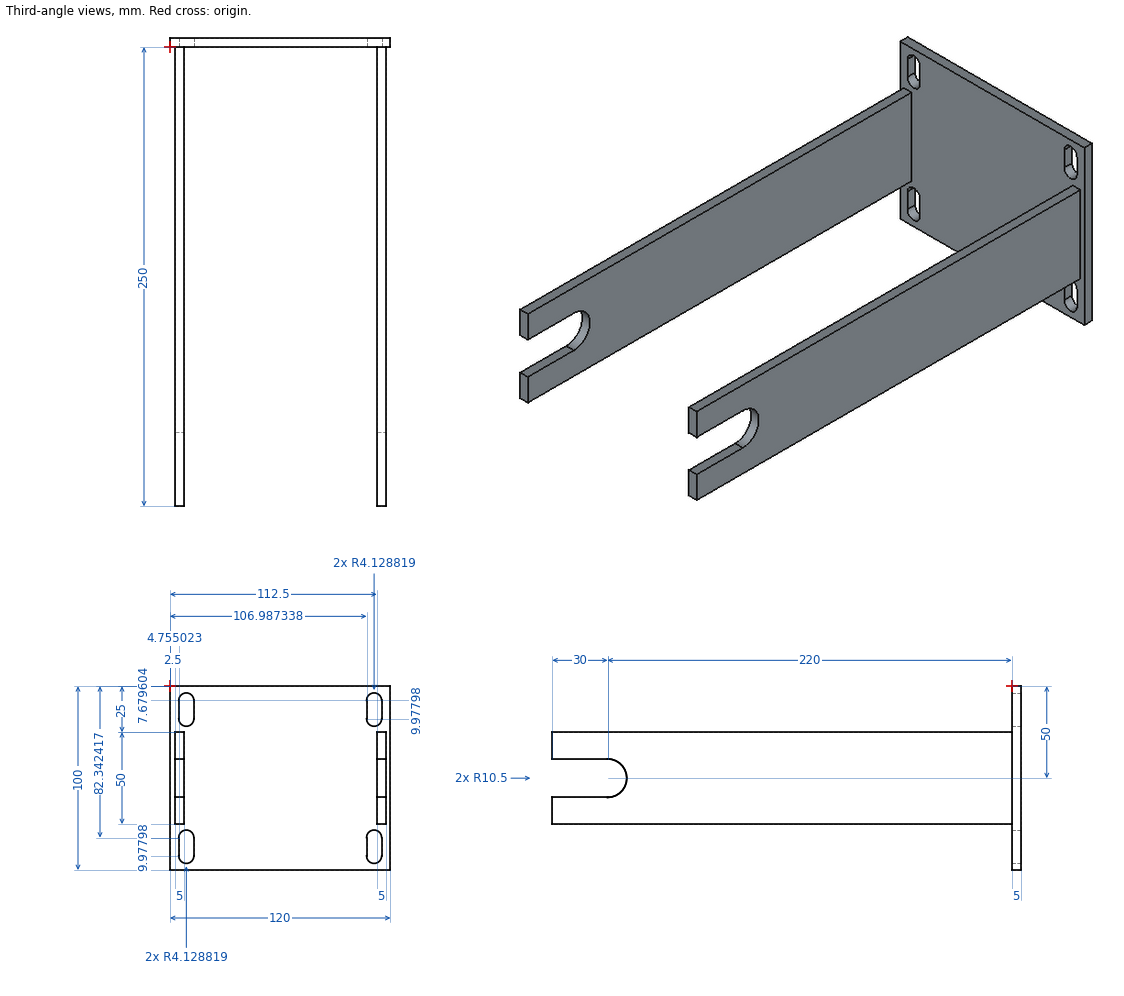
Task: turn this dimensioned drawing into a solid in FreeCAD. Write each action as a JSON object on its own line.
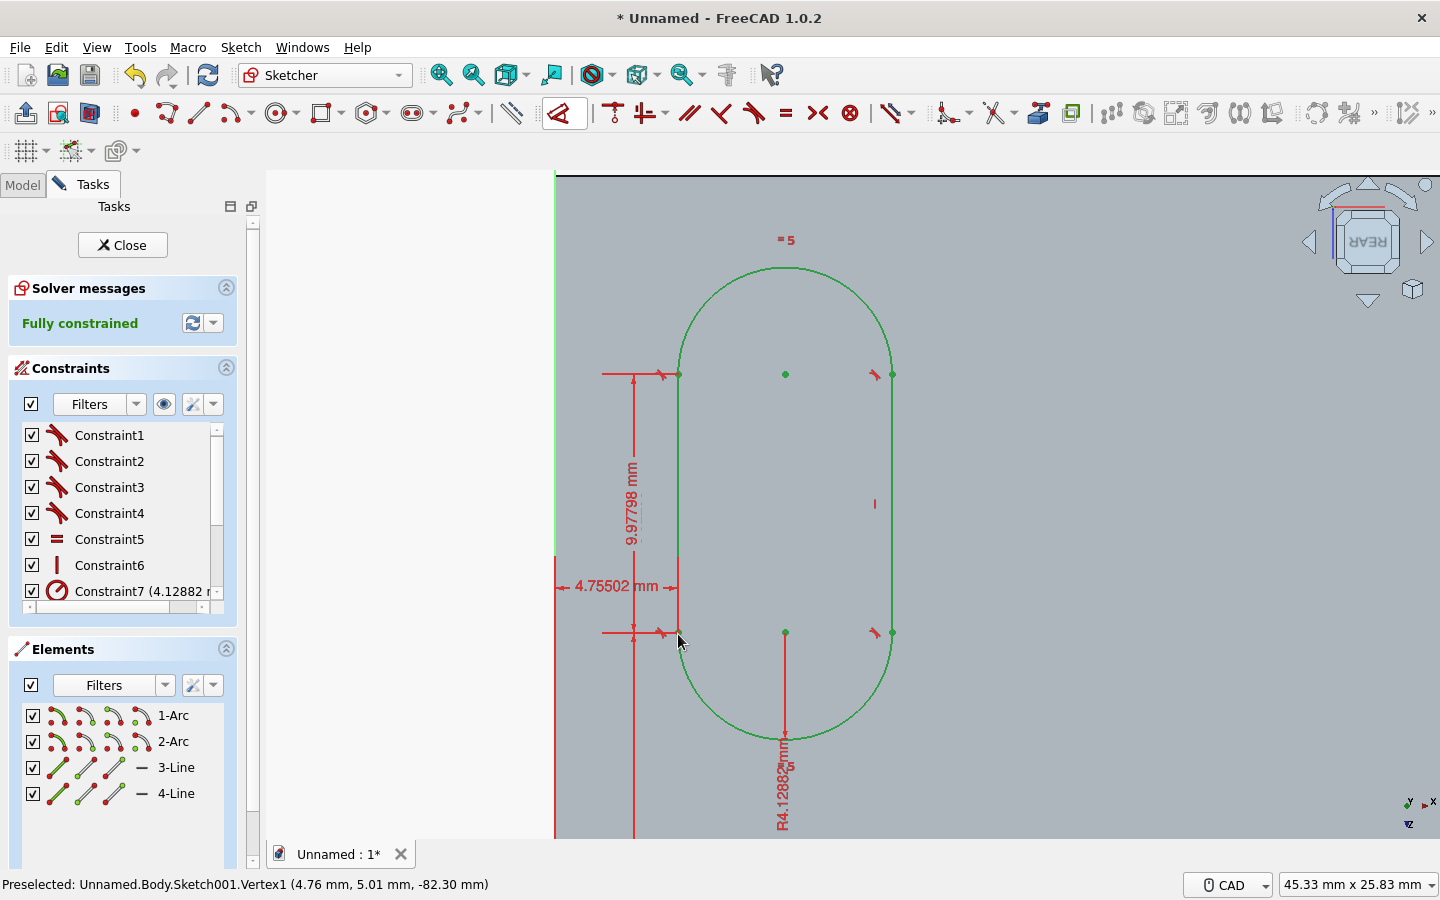
{"action": "left_click", "coordinate": [123, 245]}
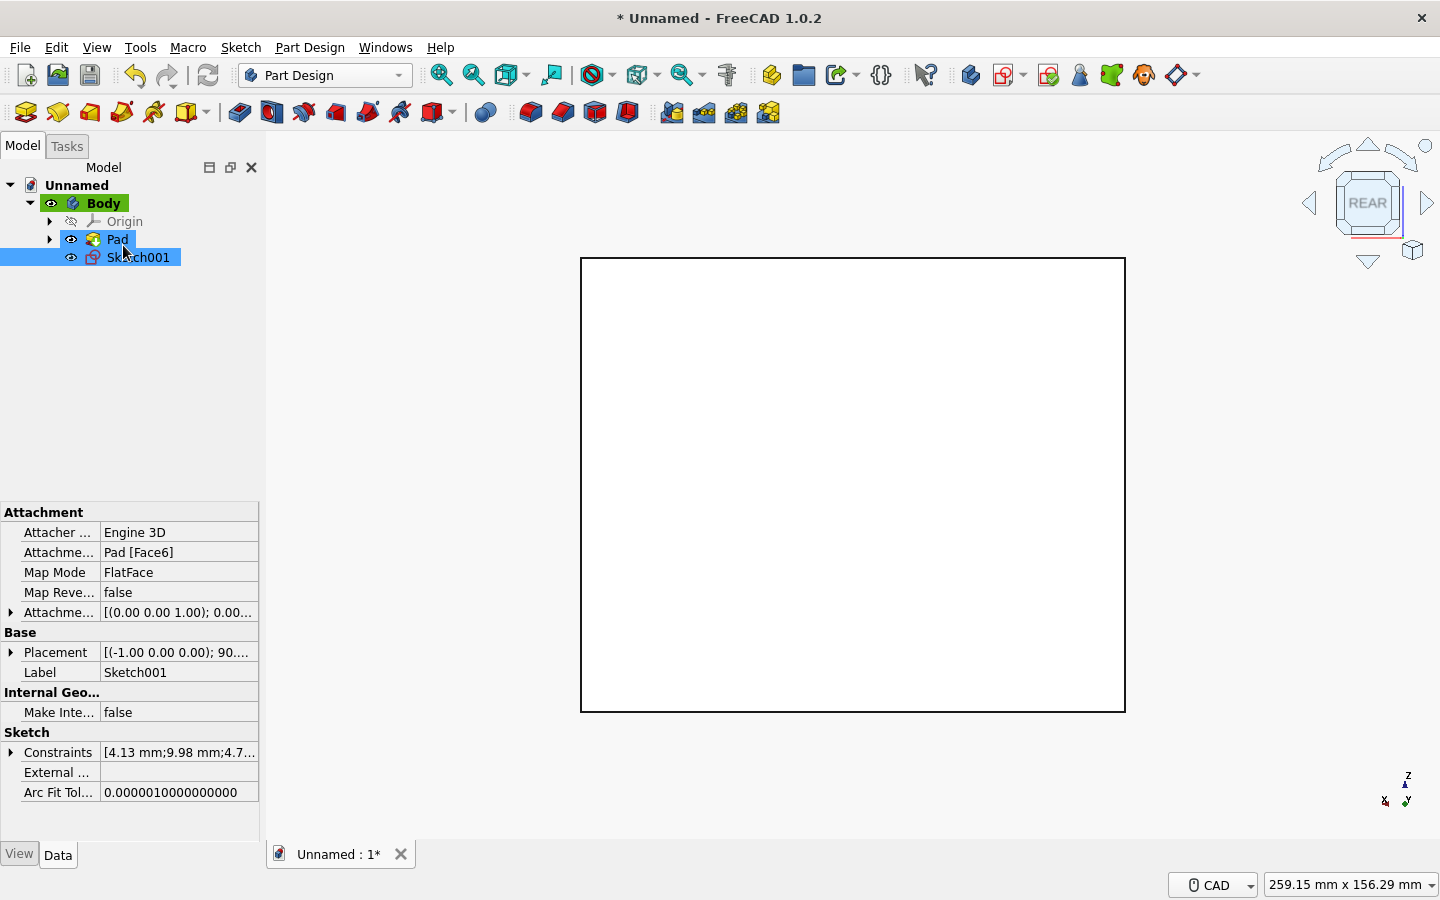
{"action": "left_click", "coordinate": [240, 112]}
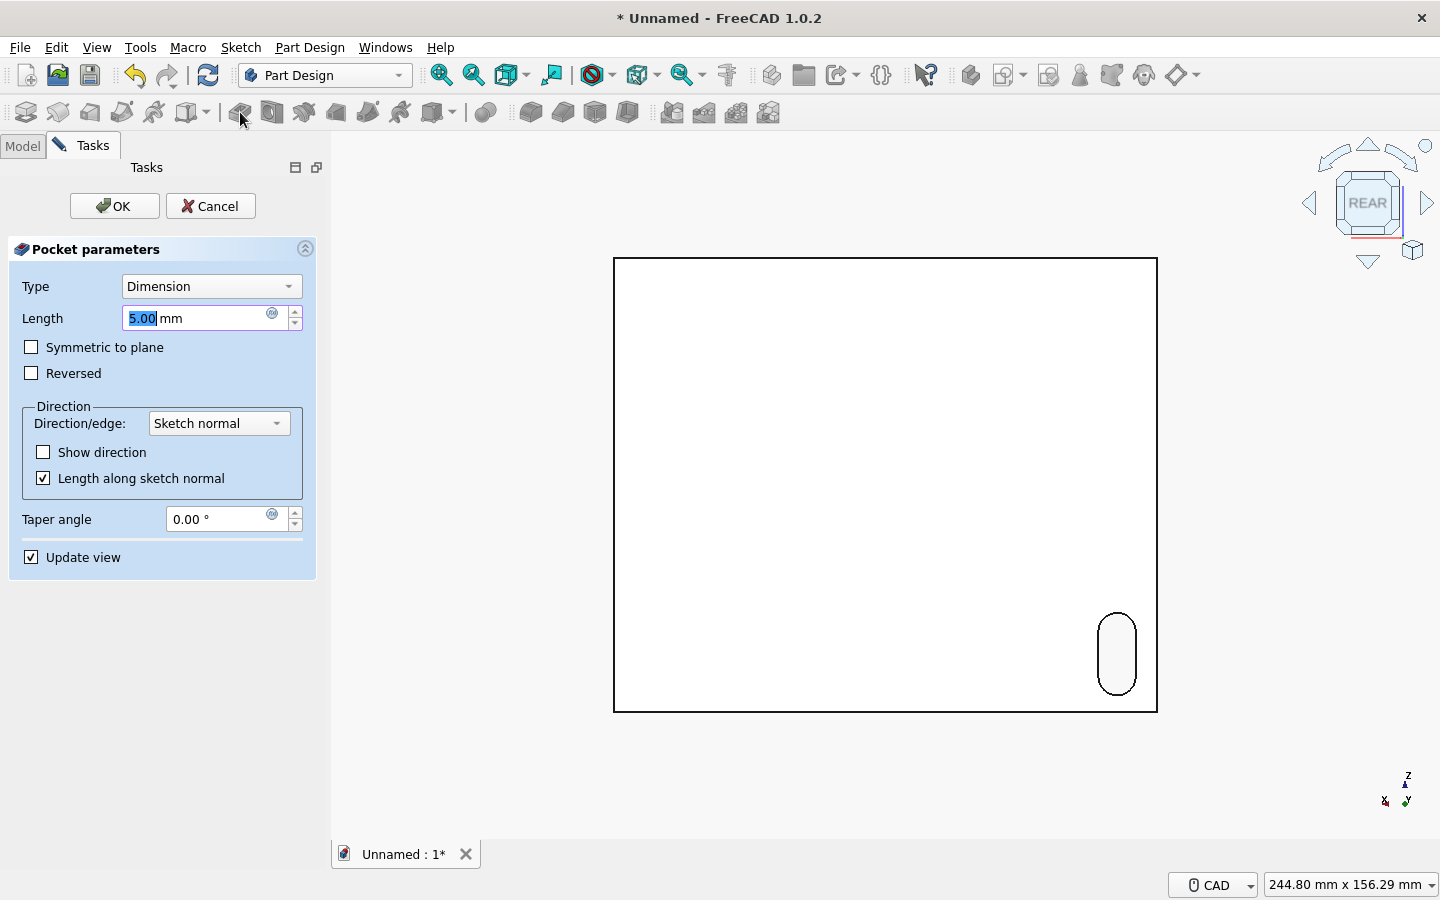
{"action": "left_click", "coordinate": [212, 286]}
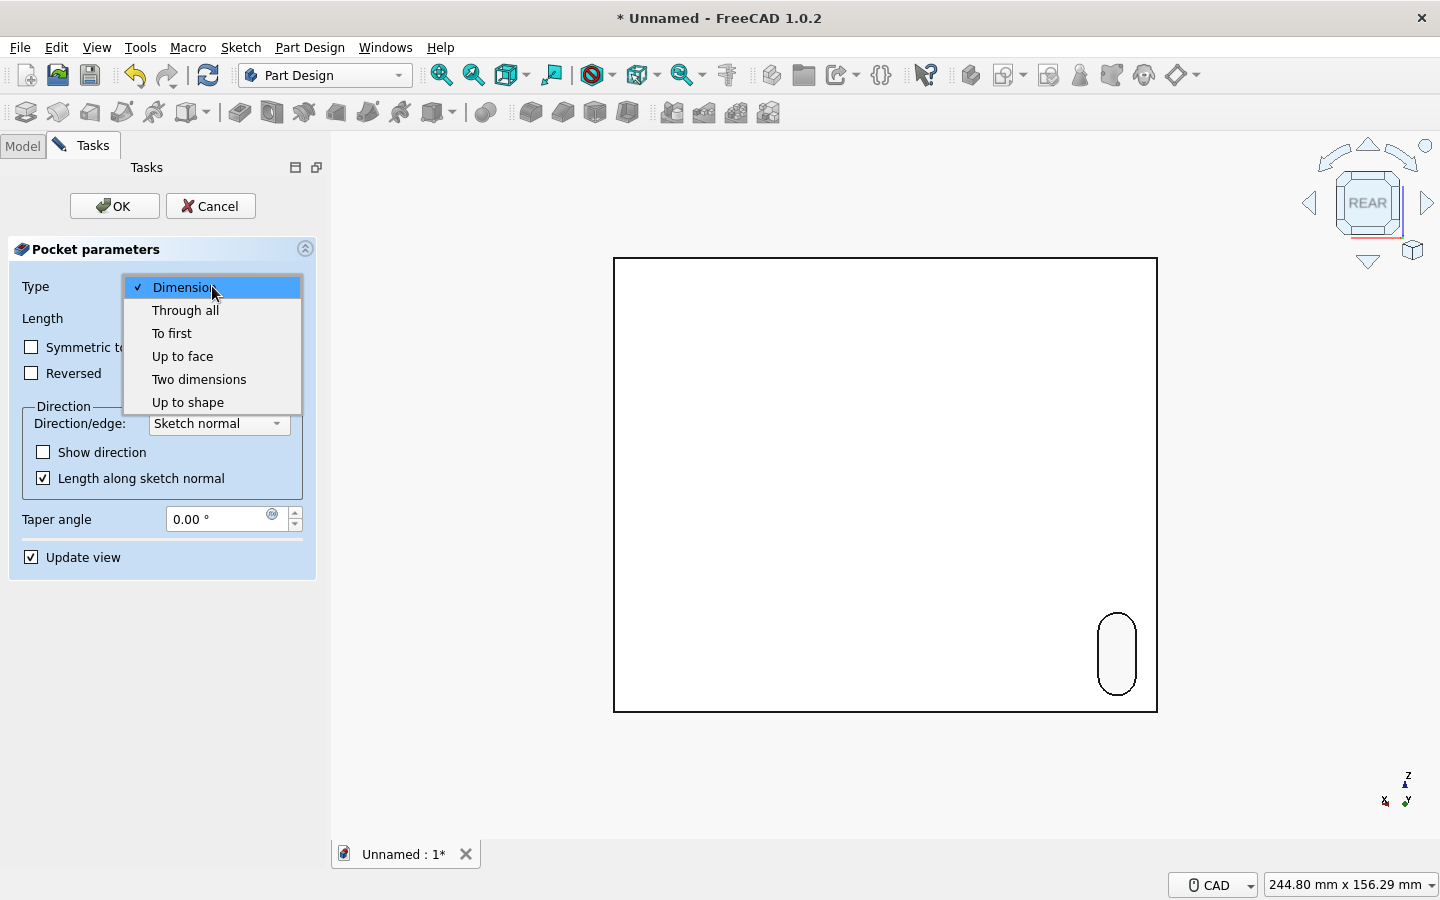
{"action": "left_click", "coordinate": [212, 310]}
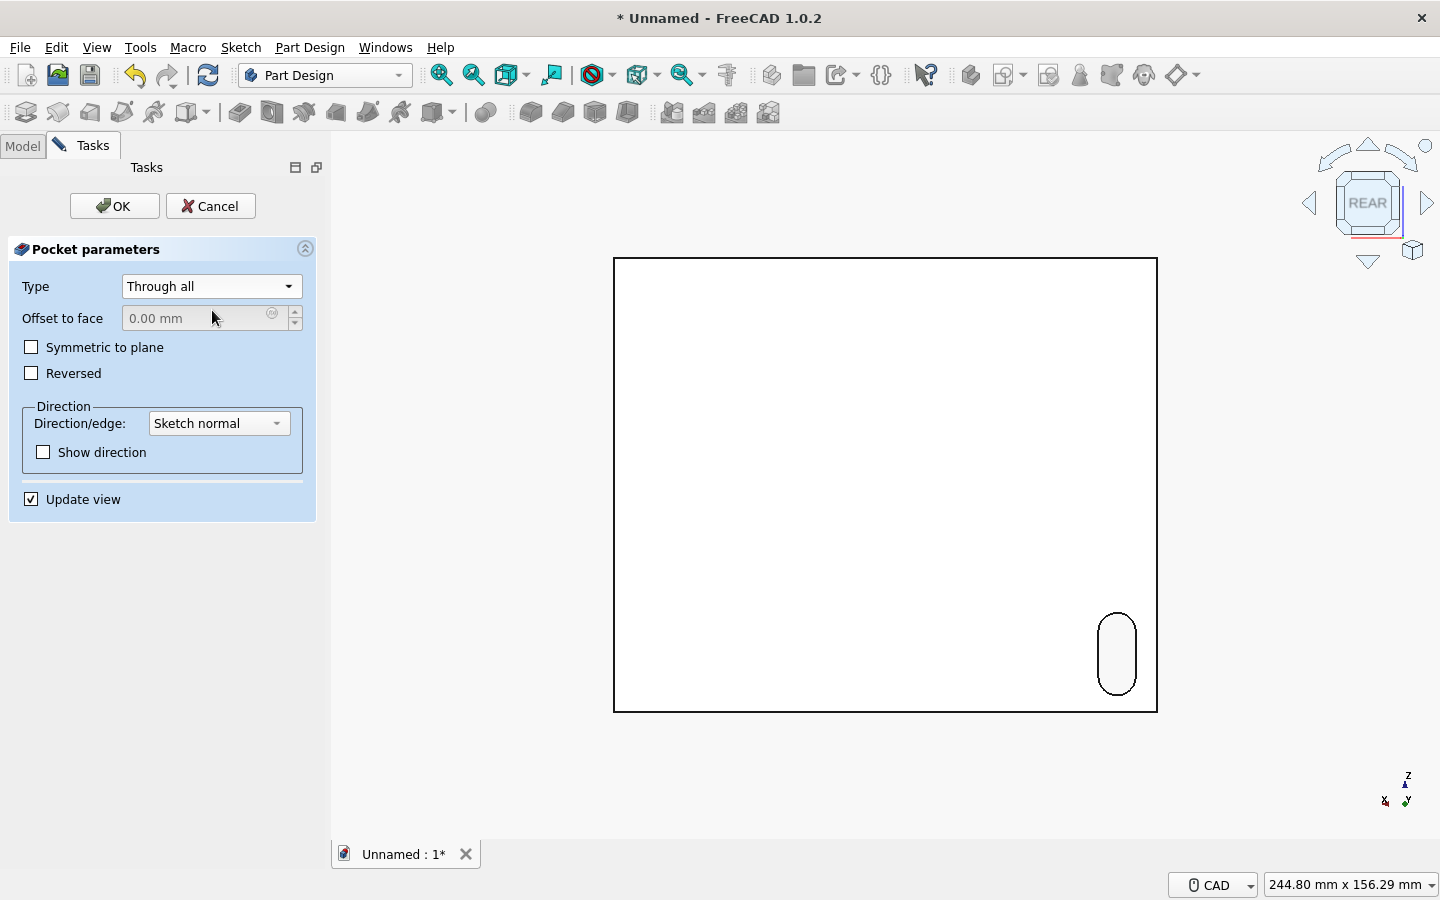
{"action": "left_click", "coordinate": [115, 206]}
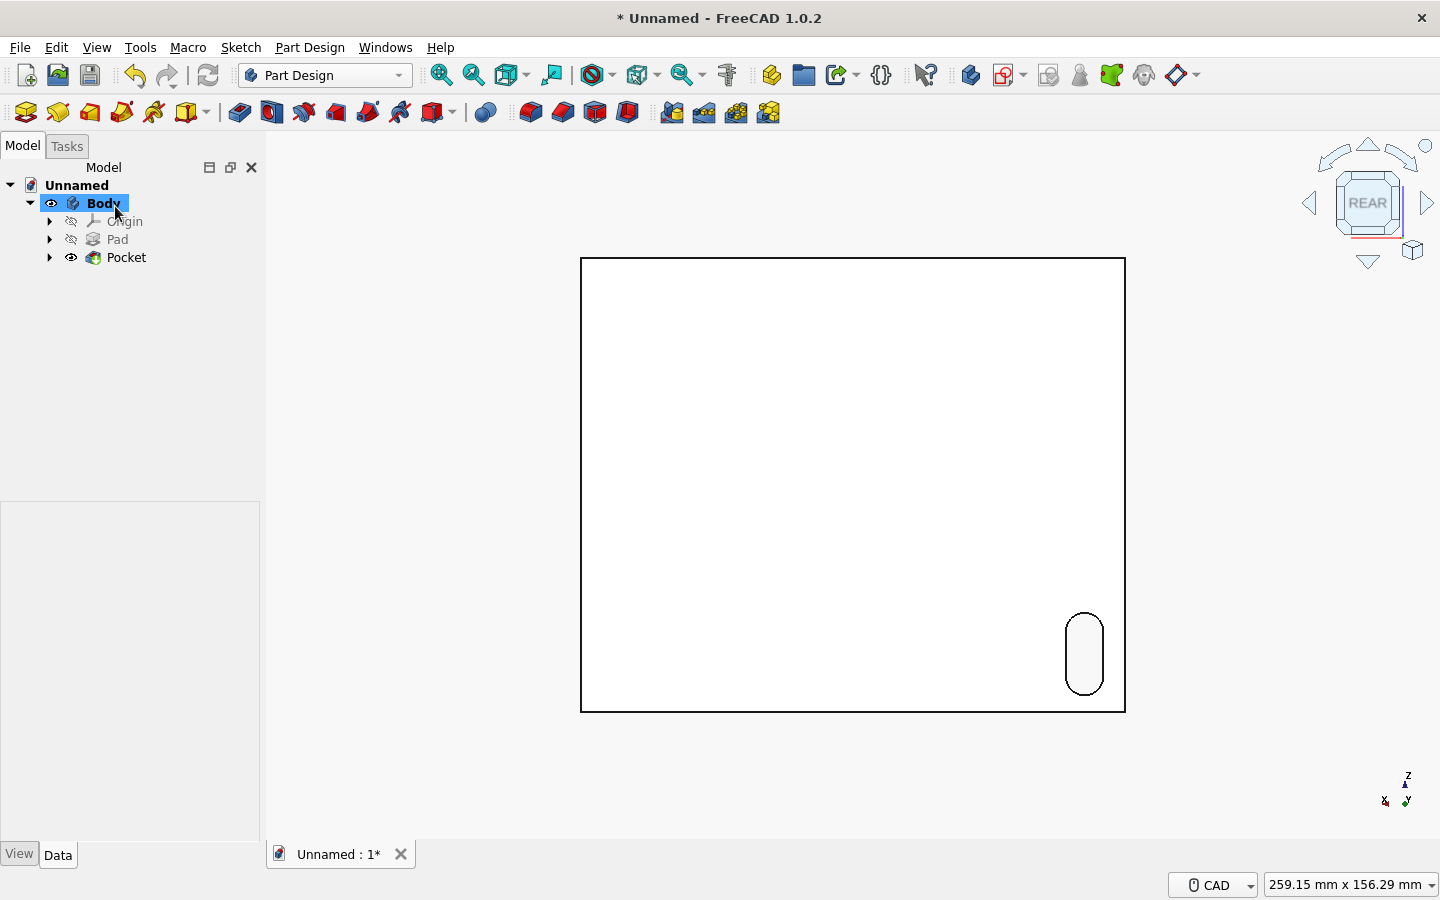
{"action": "left_click", "coordinate": [50, 221]}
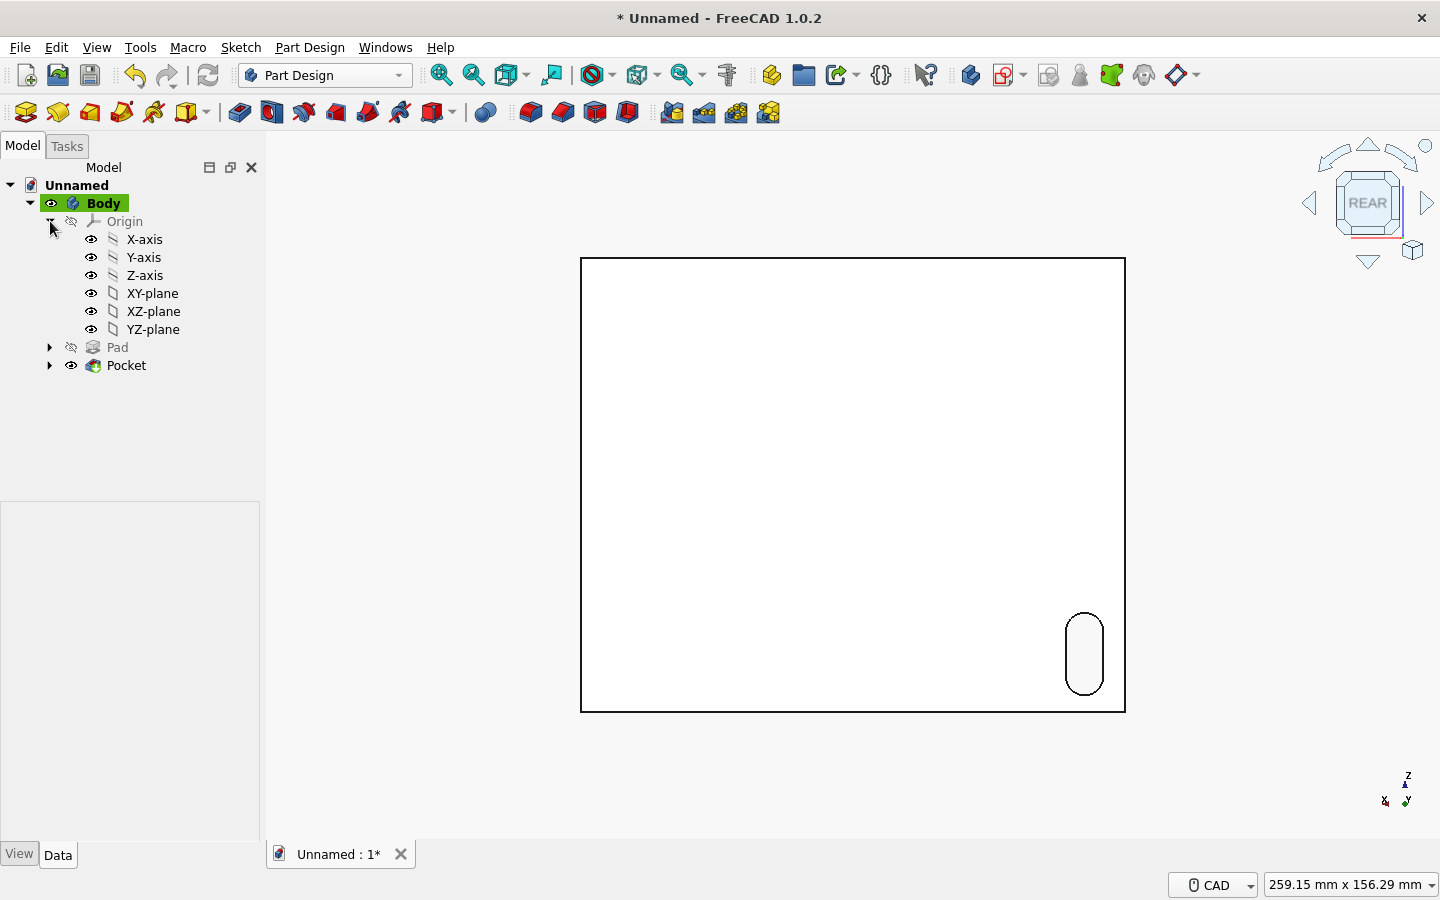
{"action": "left_click", "coordinate": [136, 329]}